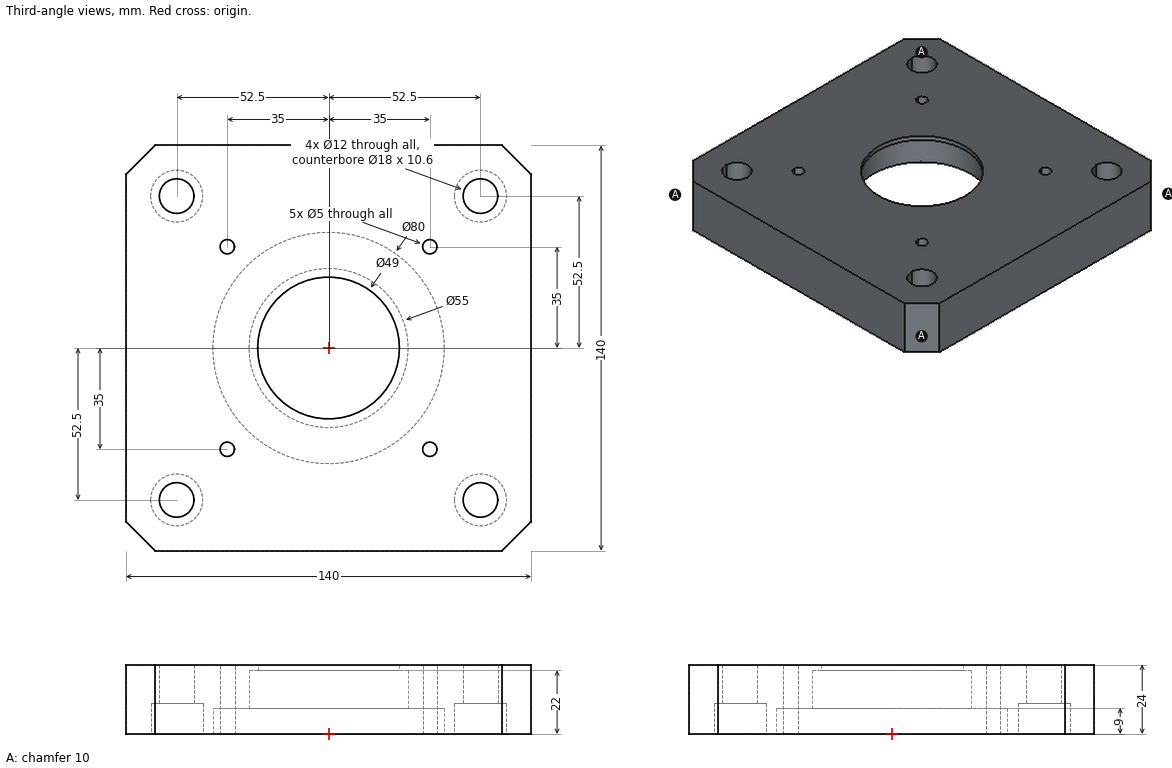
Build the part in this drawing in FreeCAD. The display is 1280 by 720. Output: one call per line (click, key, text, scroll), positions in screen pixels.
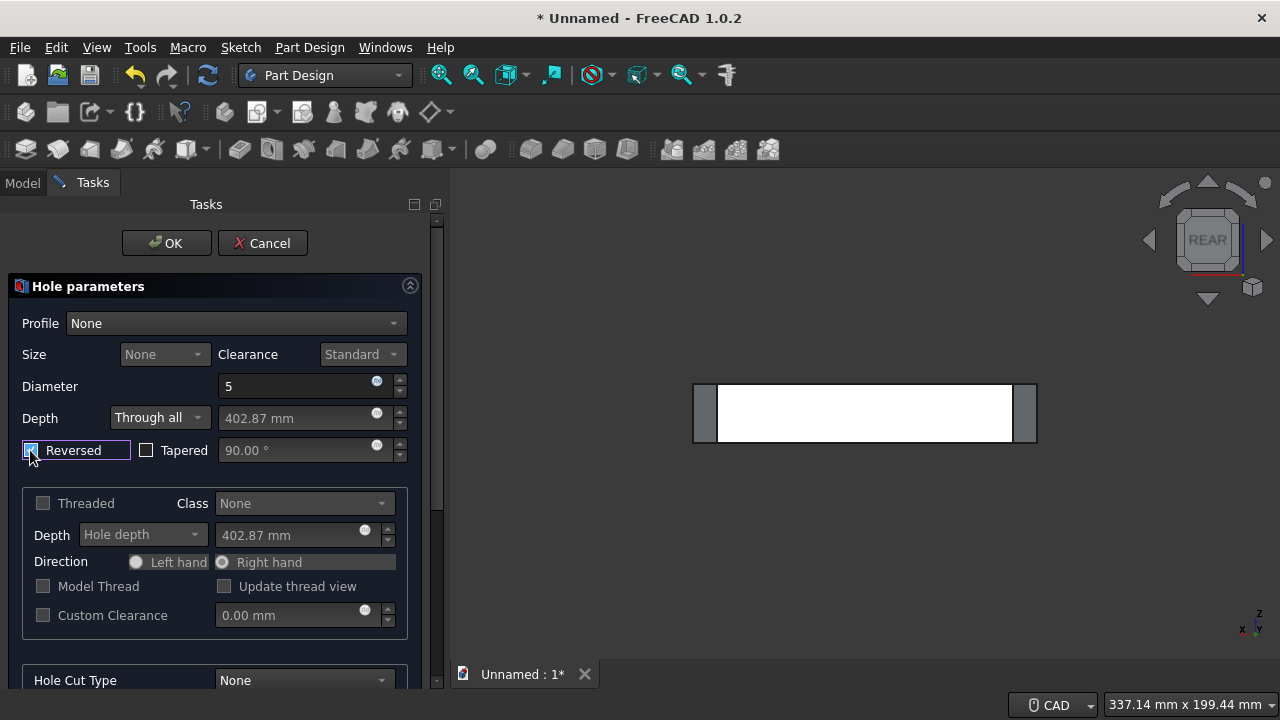
click(167, 243)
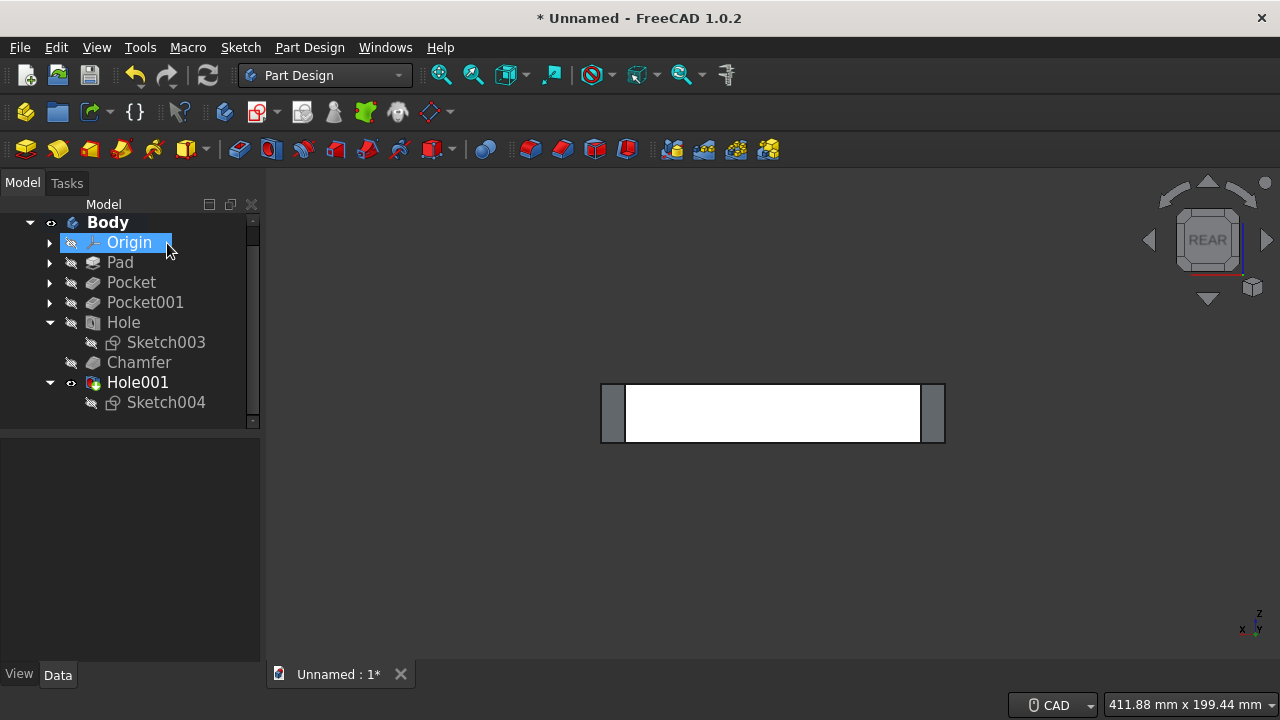
click(442, 76)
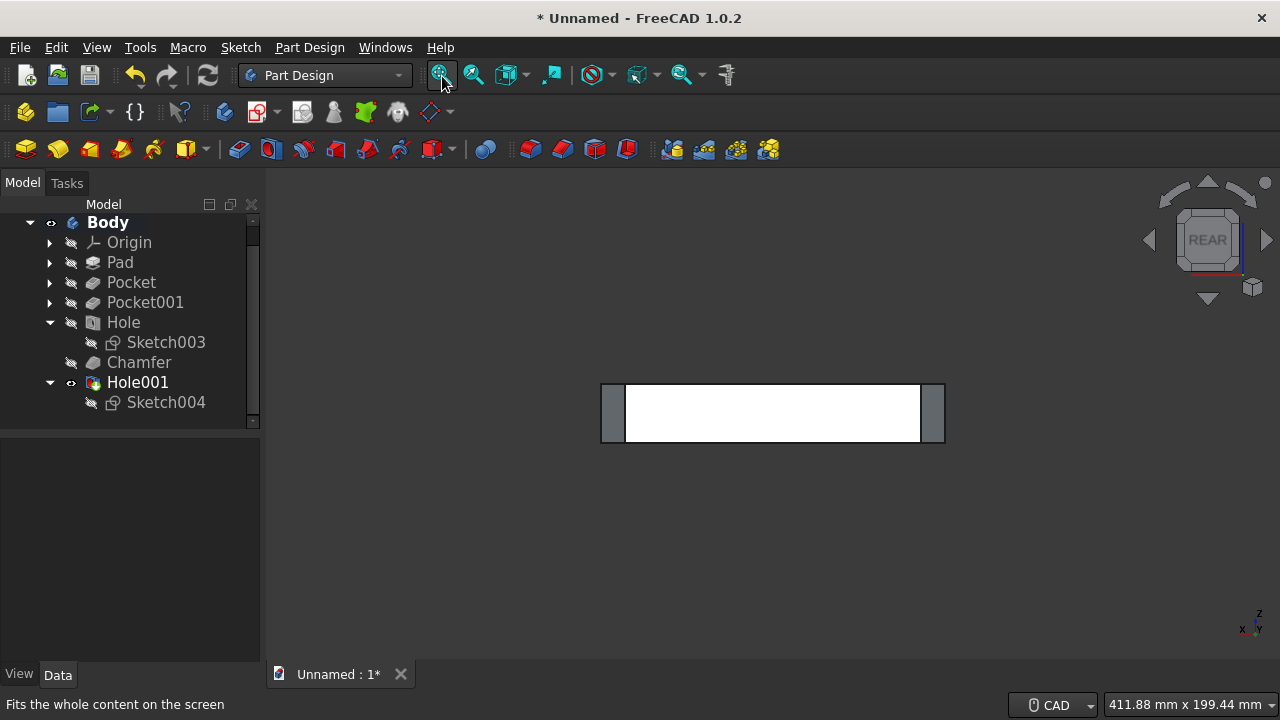
click(258, 112)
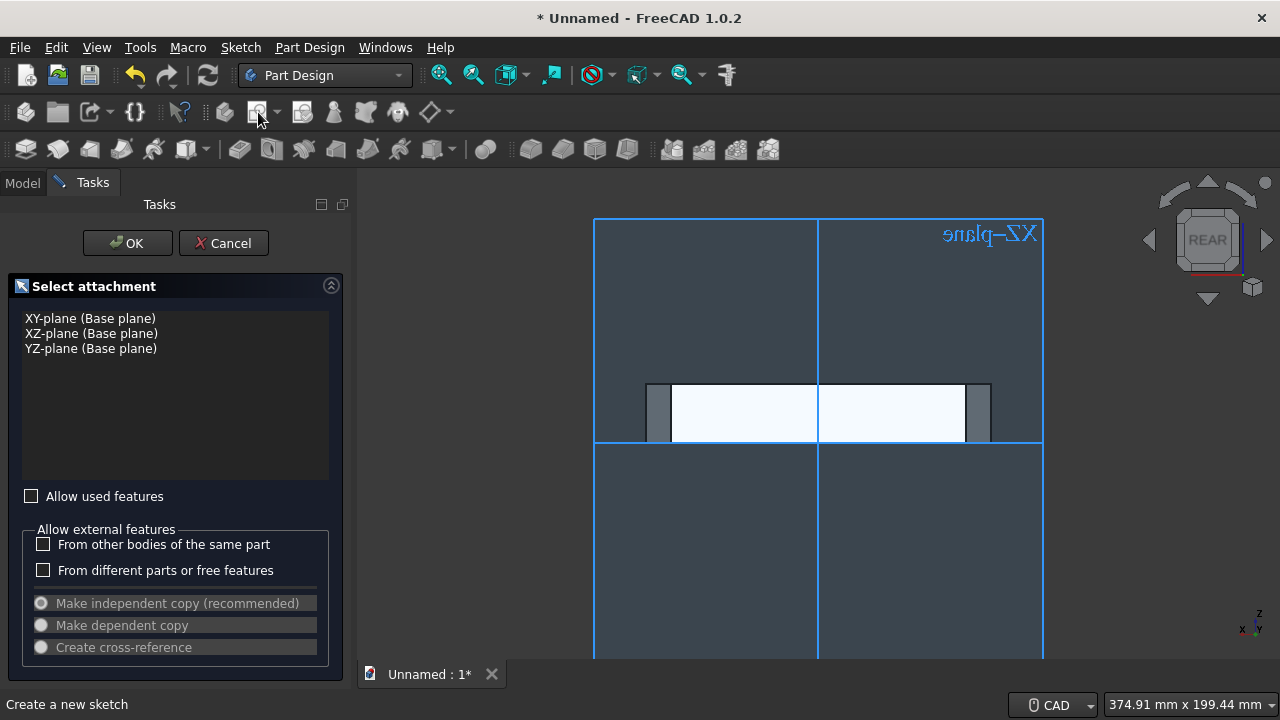
click(82, 318)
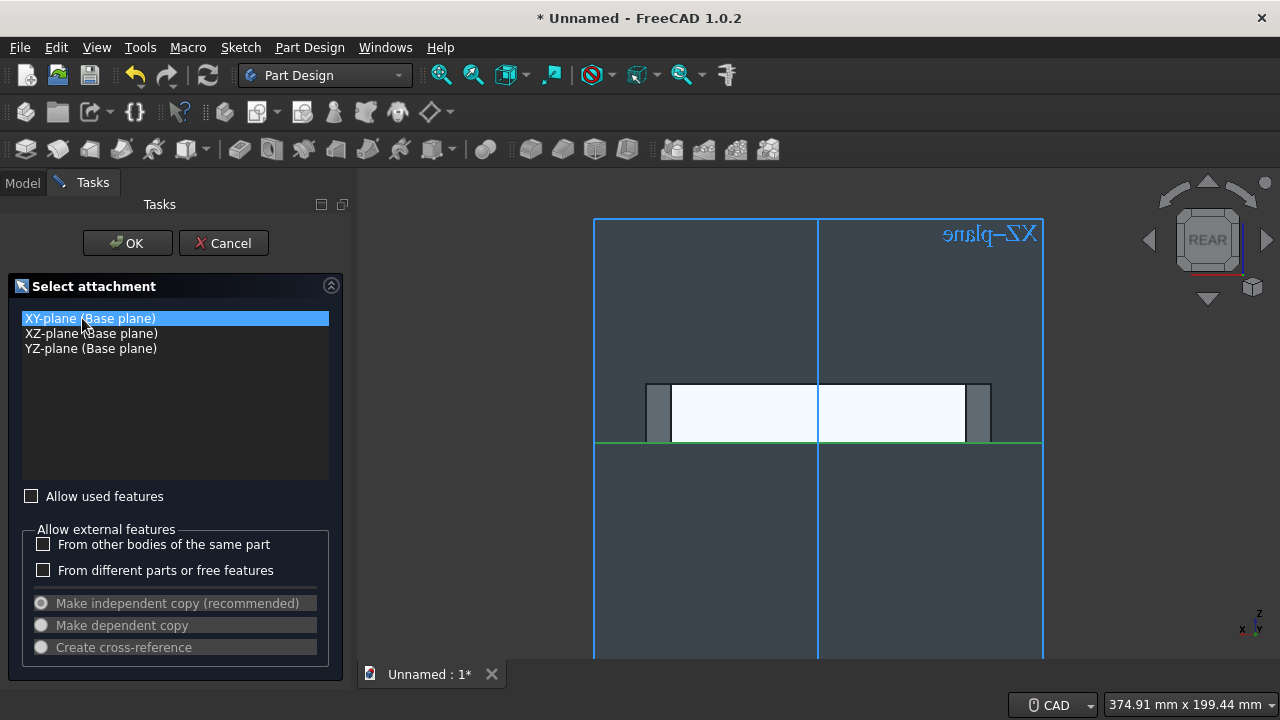
click(128, 243)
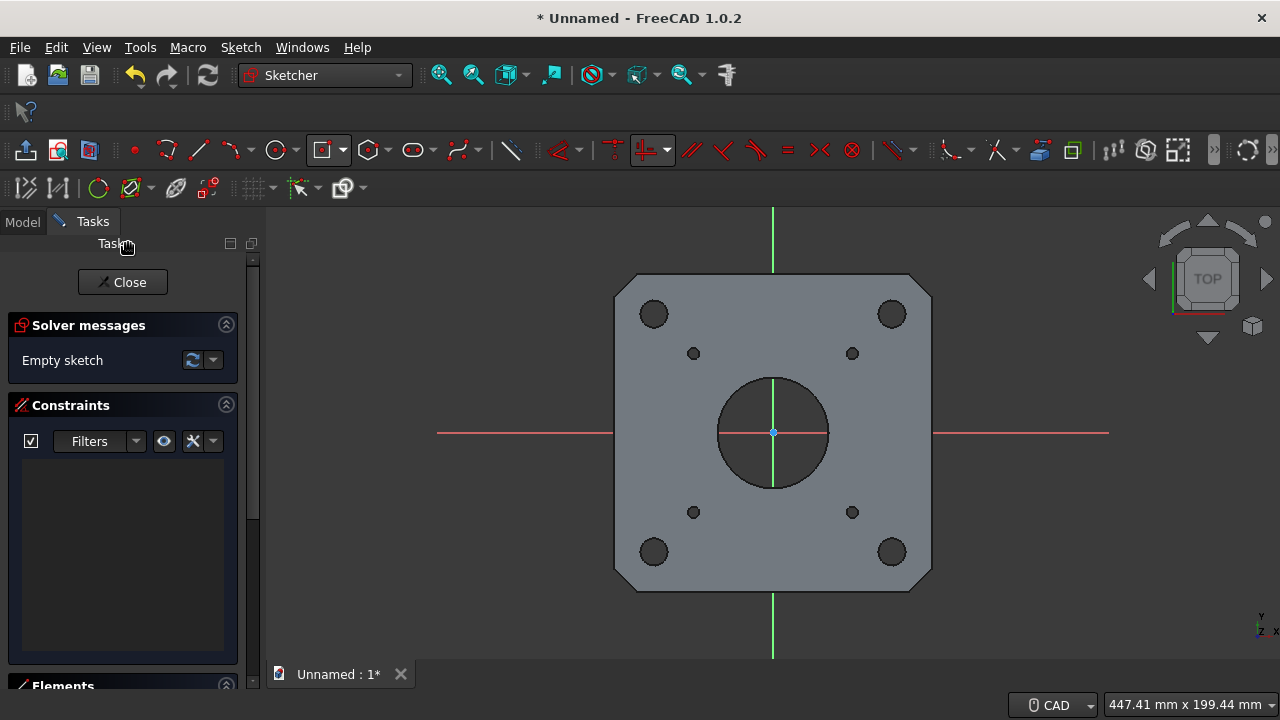
click(90, 150)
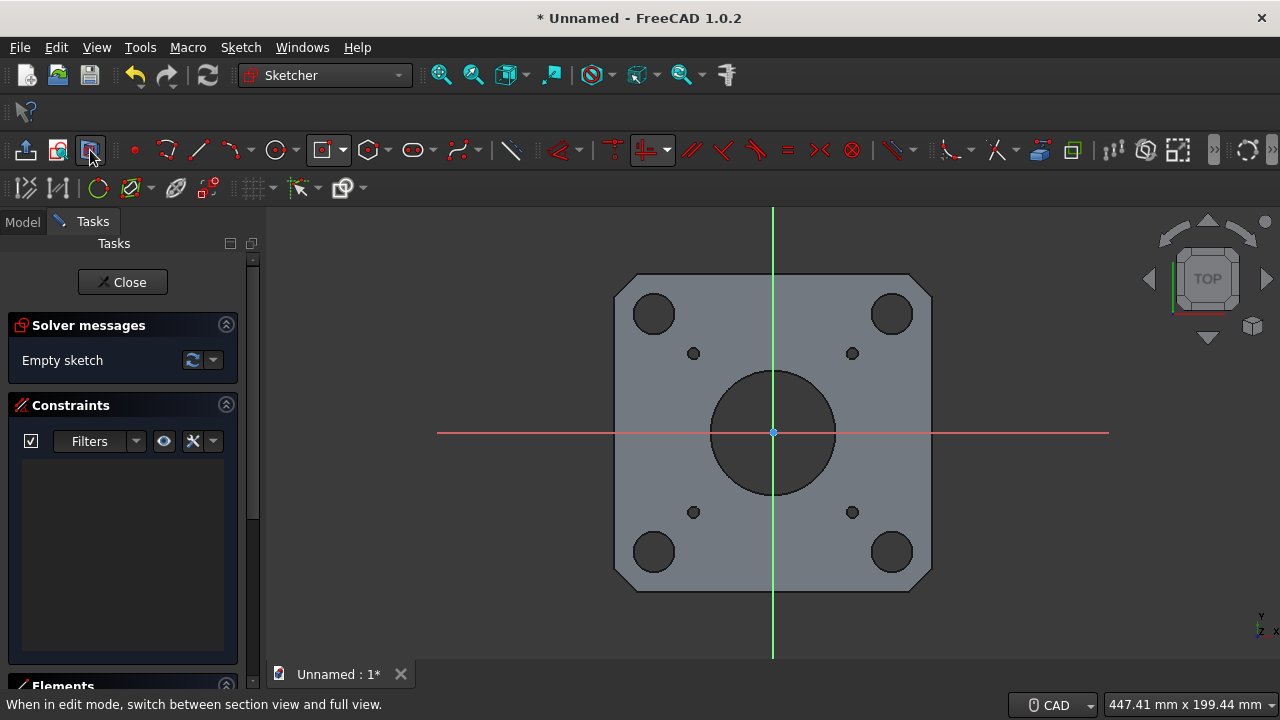
scroll(912, 433, up, 2)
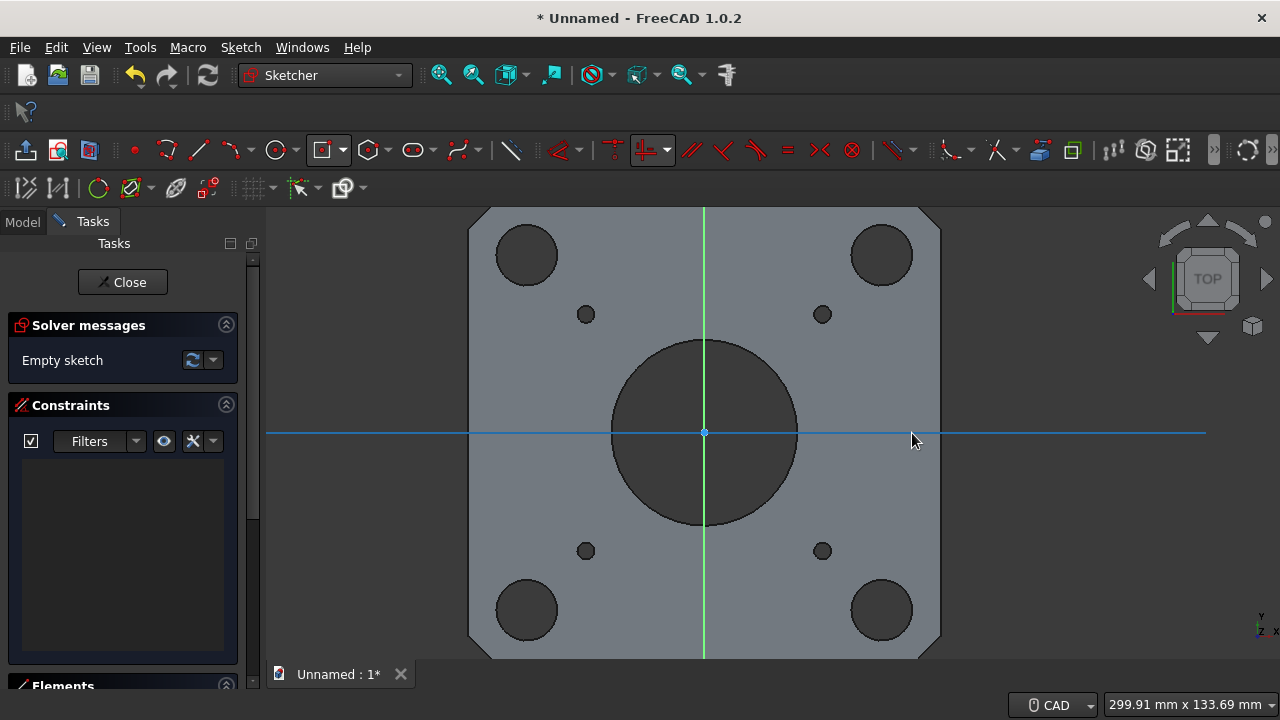
click(276, 150)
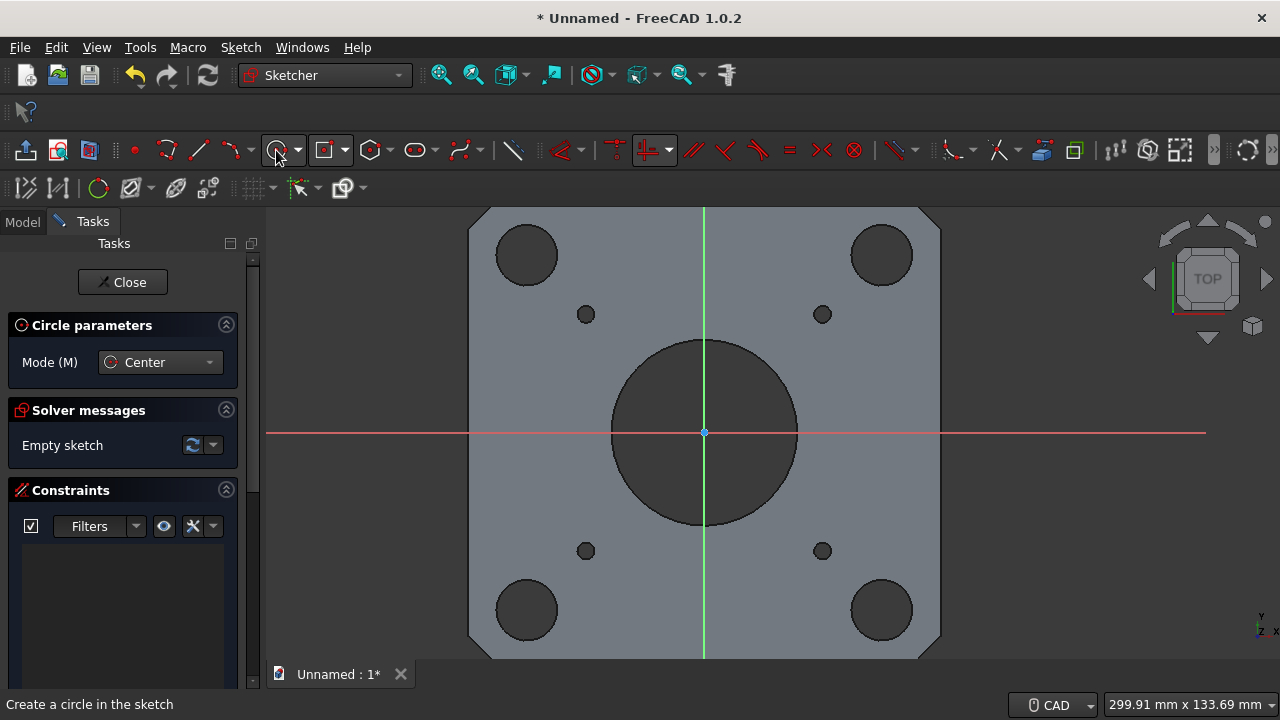
click(704, 433)
move(800, 337)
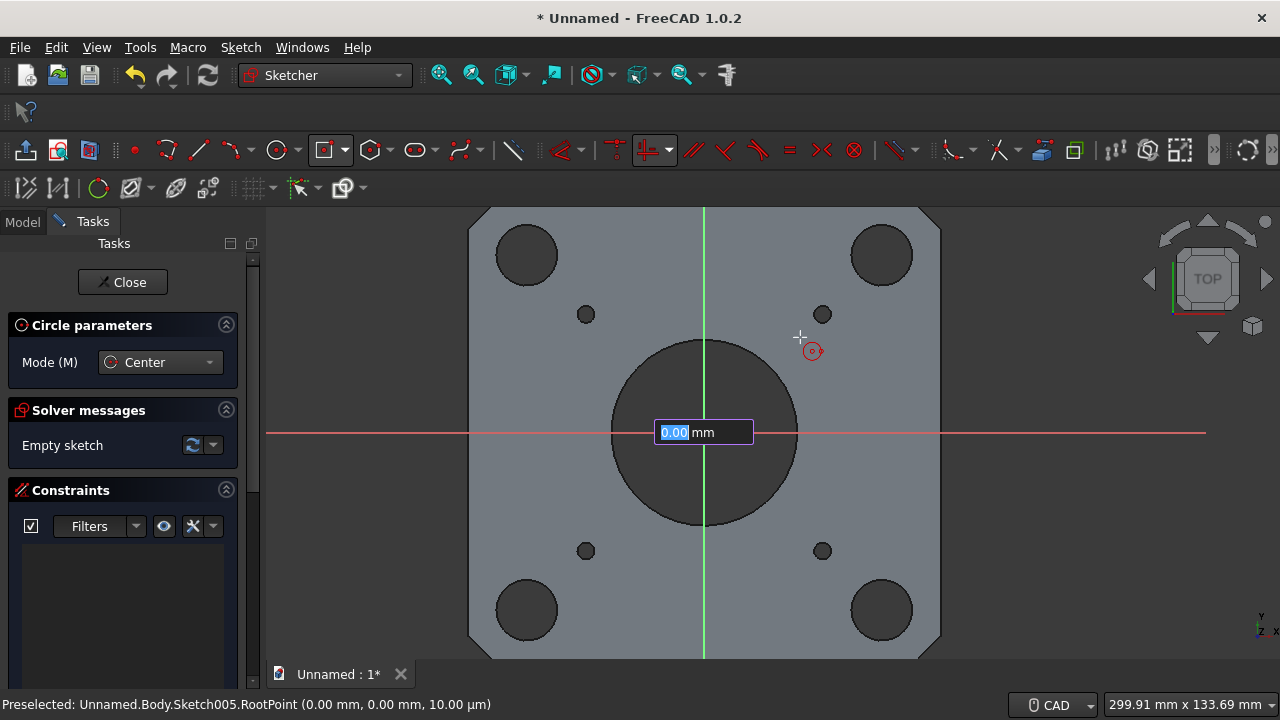
text(80)
key(Return)
key(Escape)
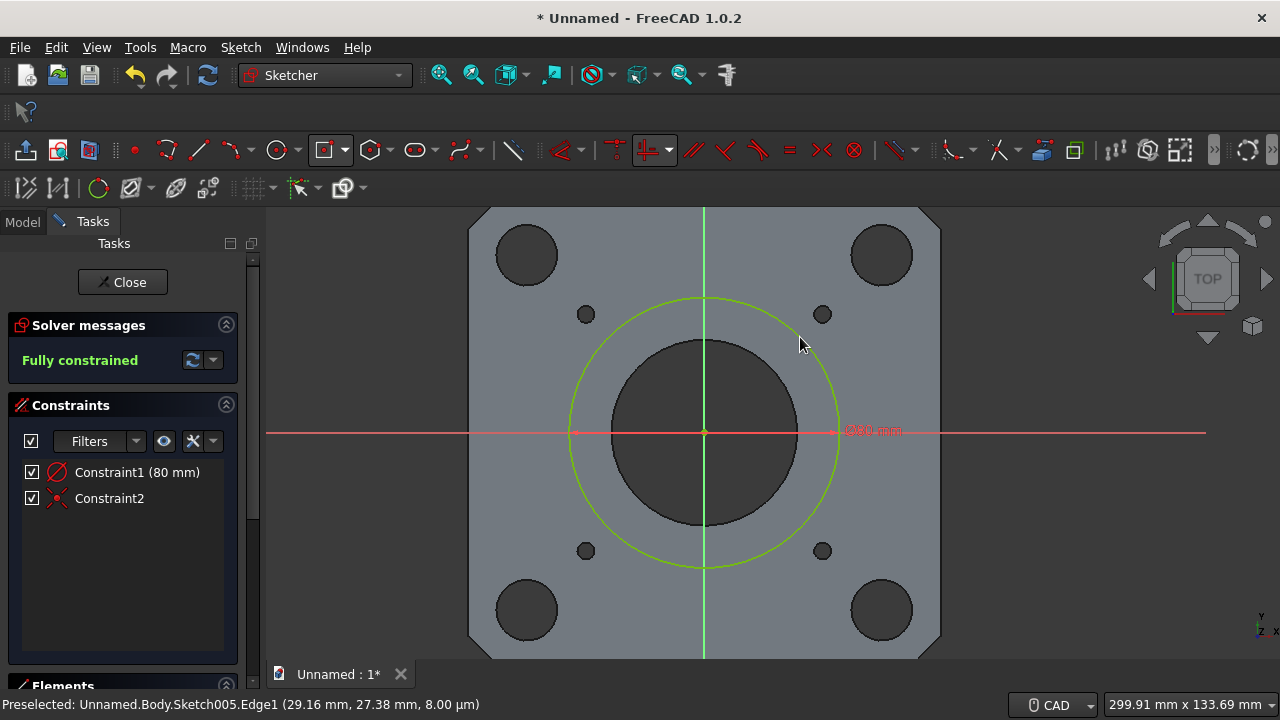
click(123, 282)